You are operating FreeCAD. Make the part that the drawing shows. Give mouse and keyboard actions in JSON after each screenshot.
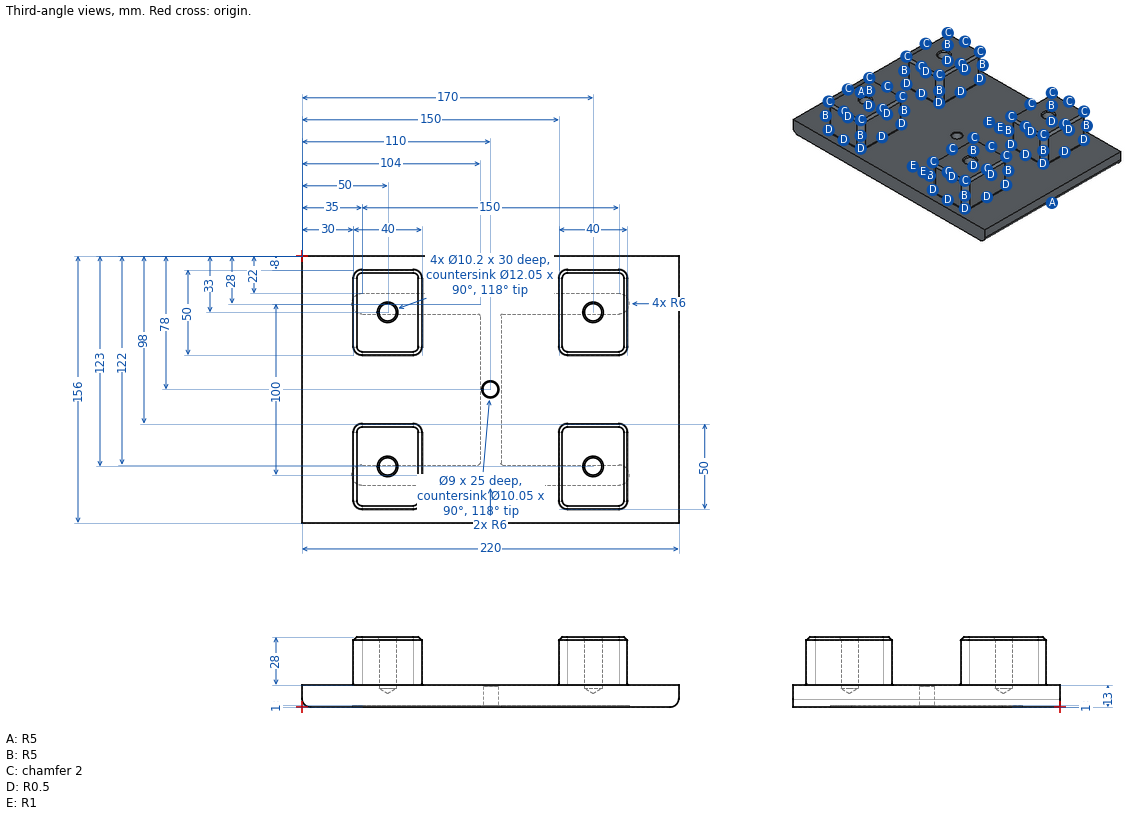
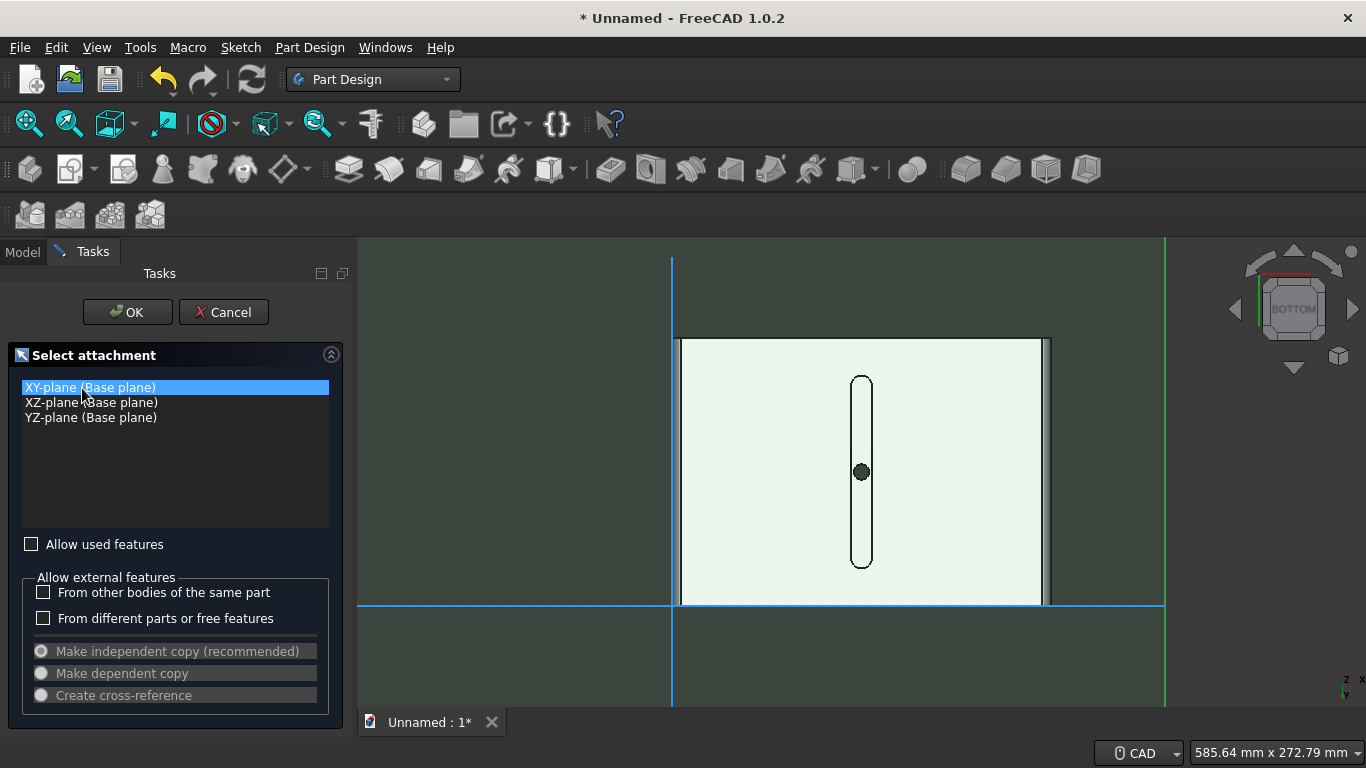
{"action": "left_click", "coordinate": [128, 312]}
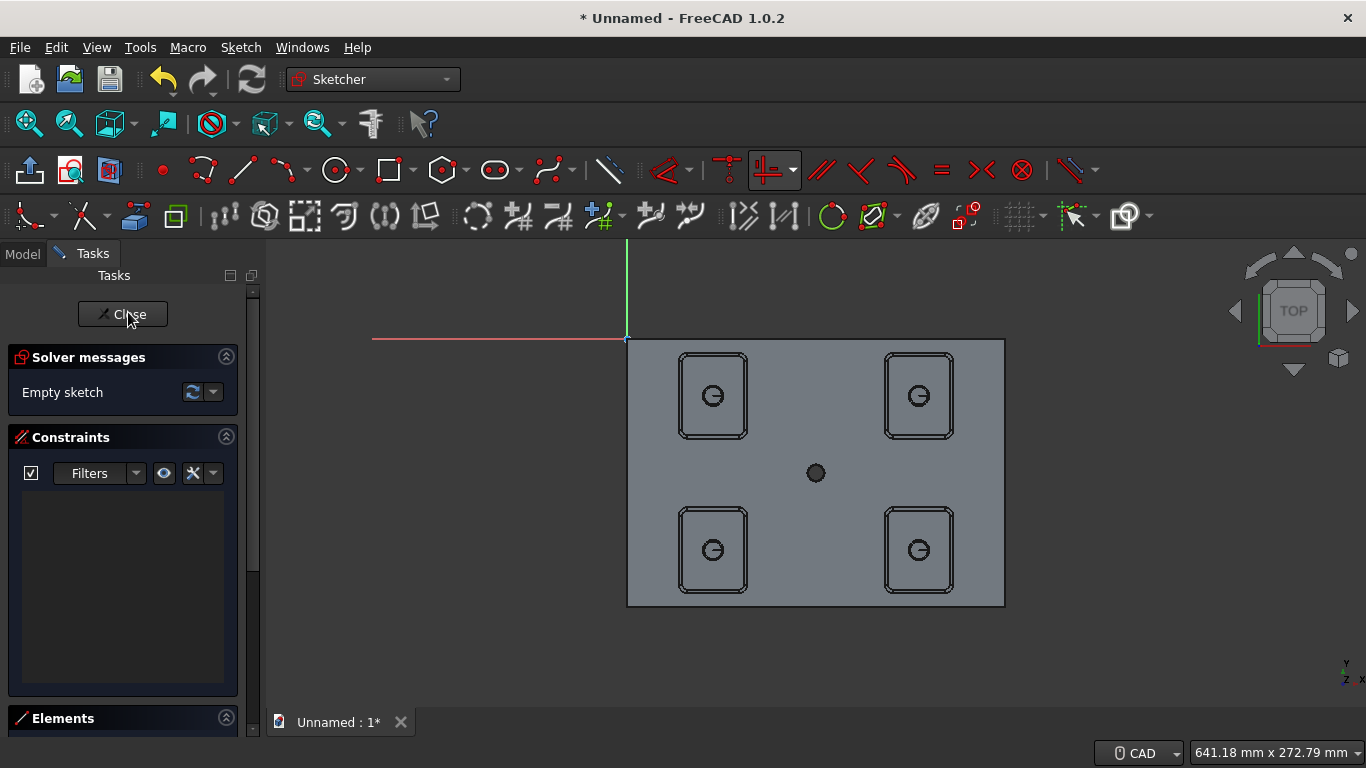
{"action": "left_click", "coordinate": [110, 170]}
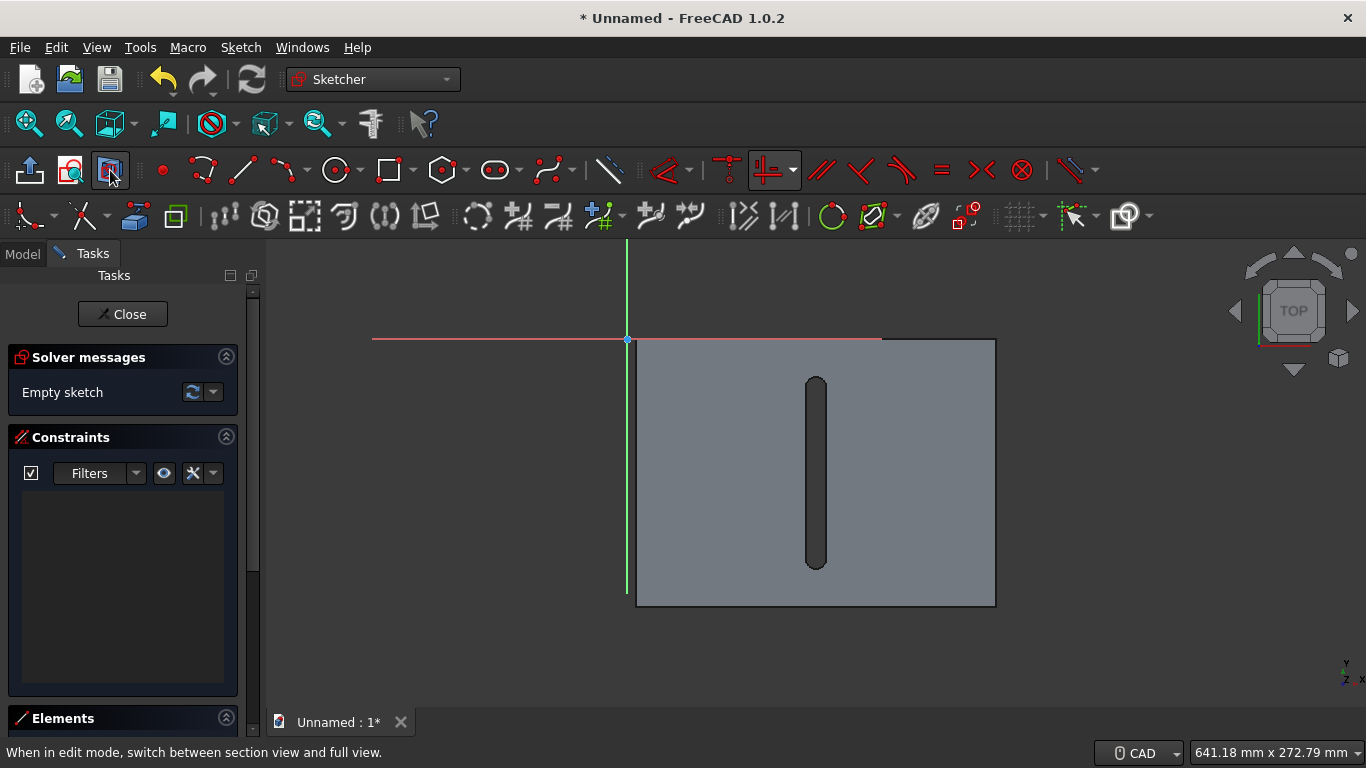
{"action": "key", "text": "g s"}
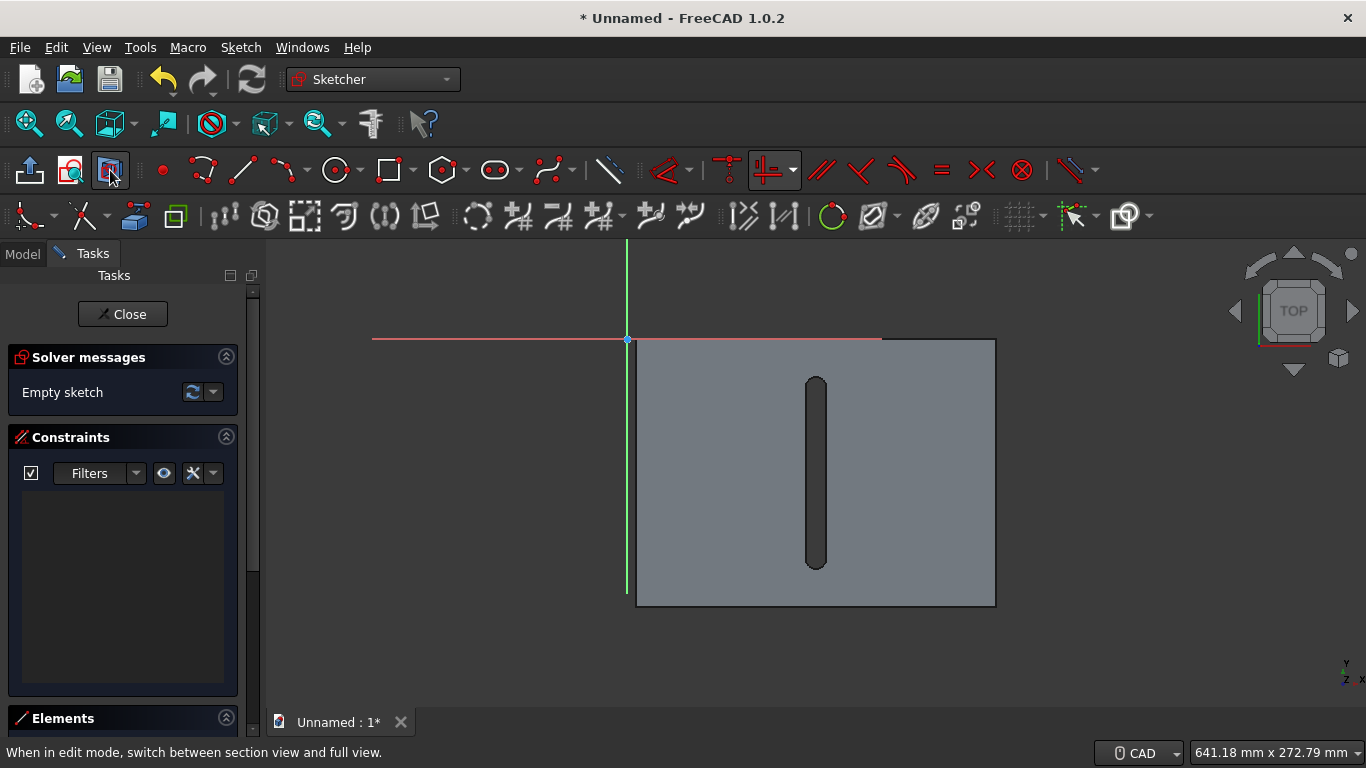
{"action": "scroll", "coordinate": [687, 387], "scroll_direction": "up", "scroll_amount": 4}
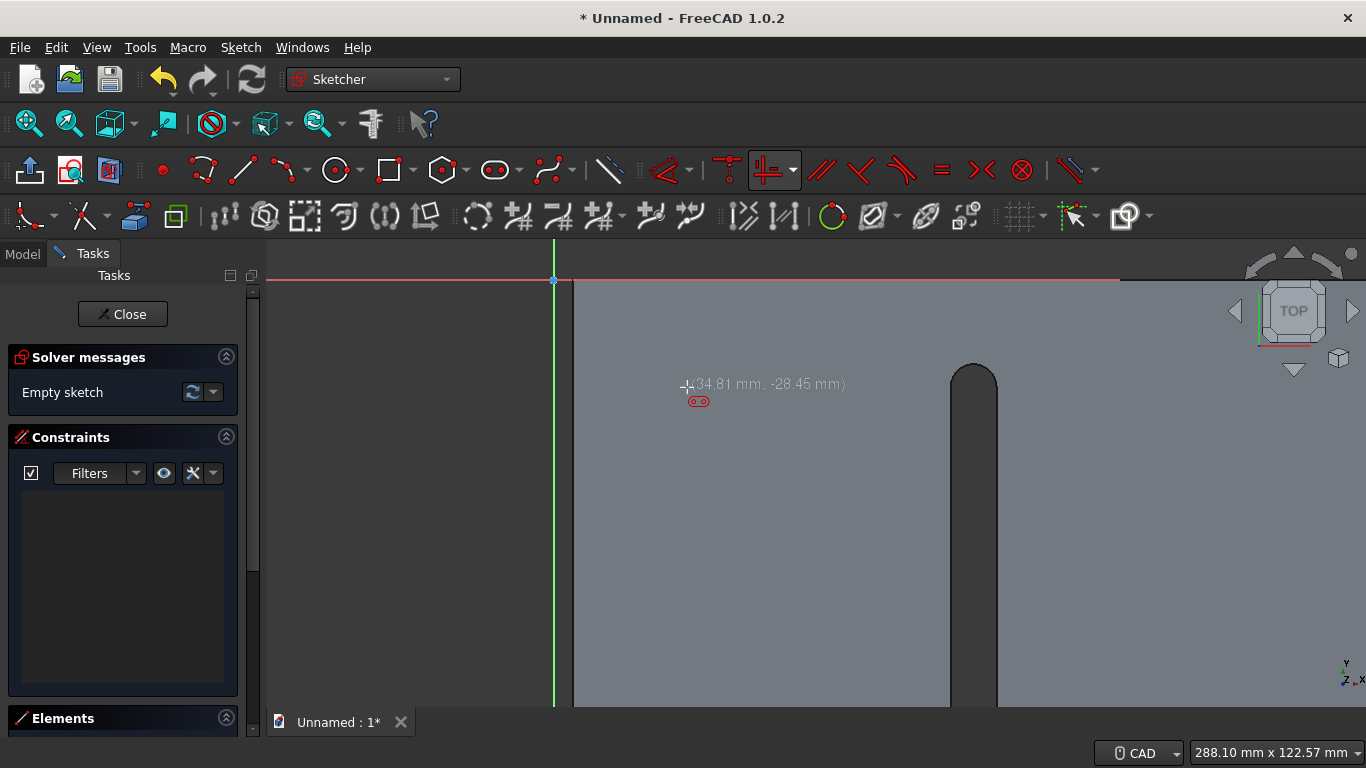
{"action": "left_click", "coordinate": [687, 387]}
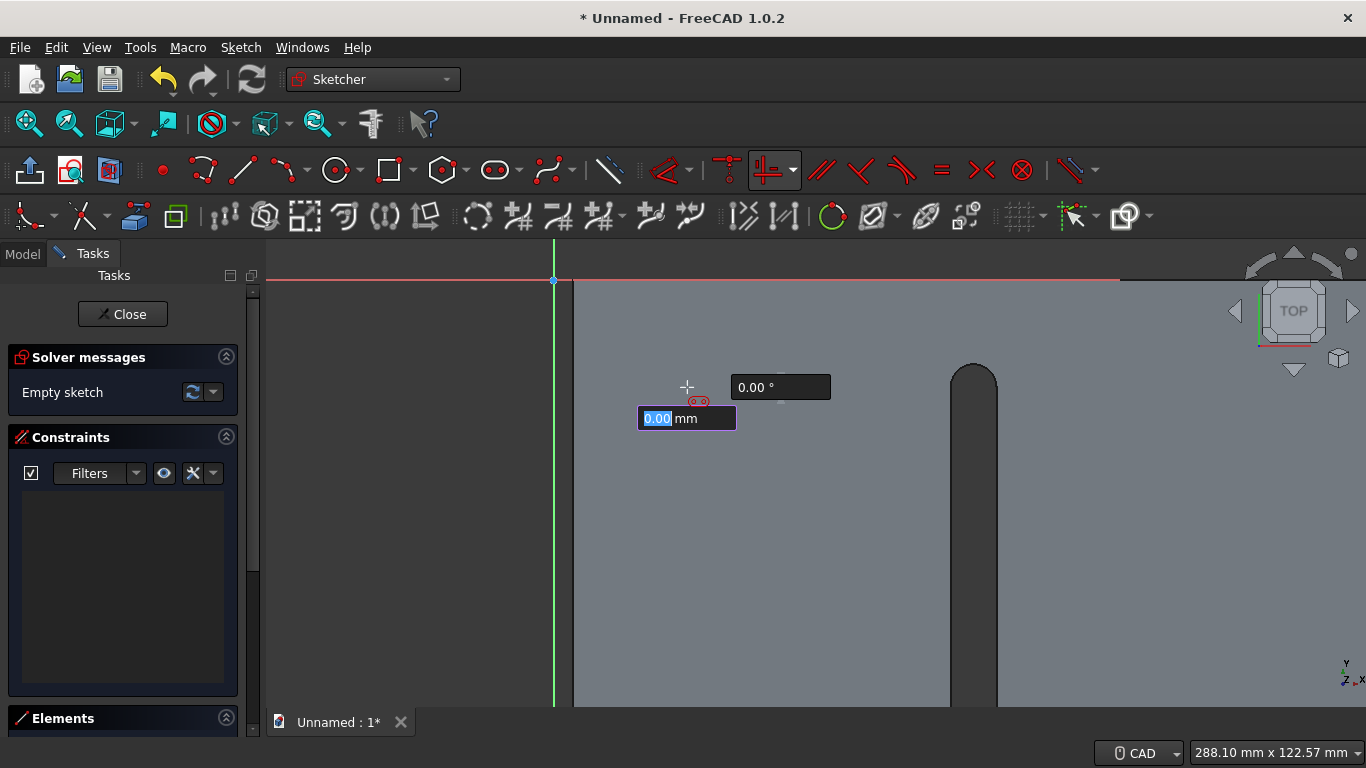
{"action": "scroll", "coordinate": [540, 396], "scroll_direction": "down", "scroll_amount": 3}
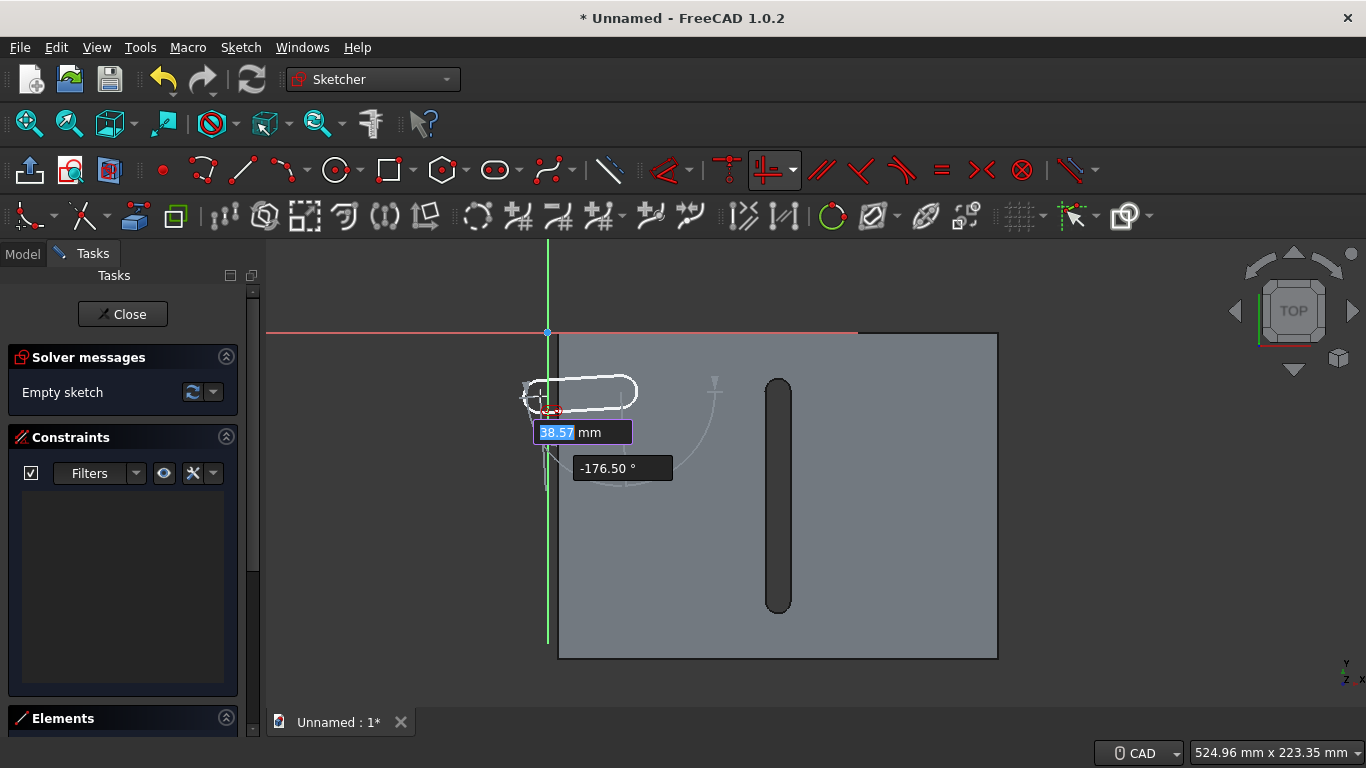
{"action": "left_click", "coordinate": [935, 391]}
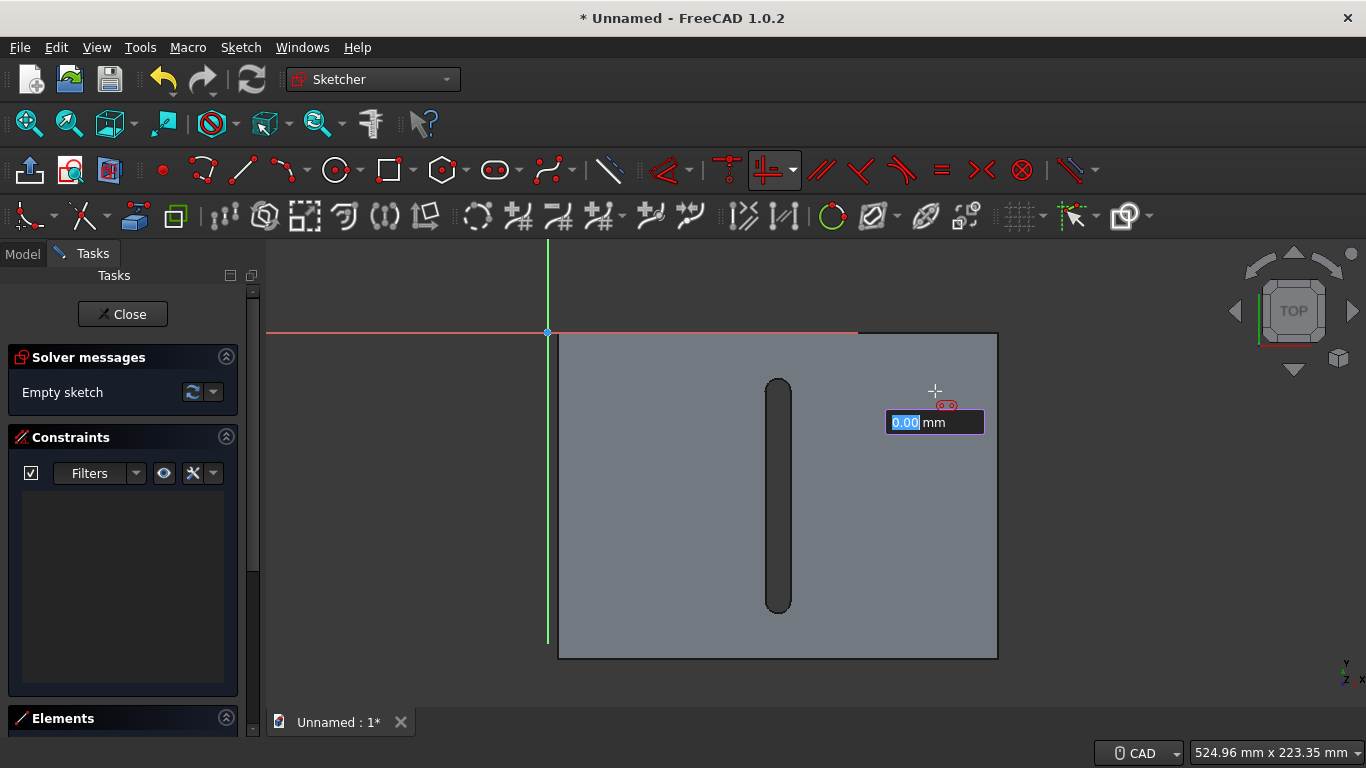
{"action": "scroll", "coordinate": [778, 379], "scroll_direction": "up", "scroll_amount": 2}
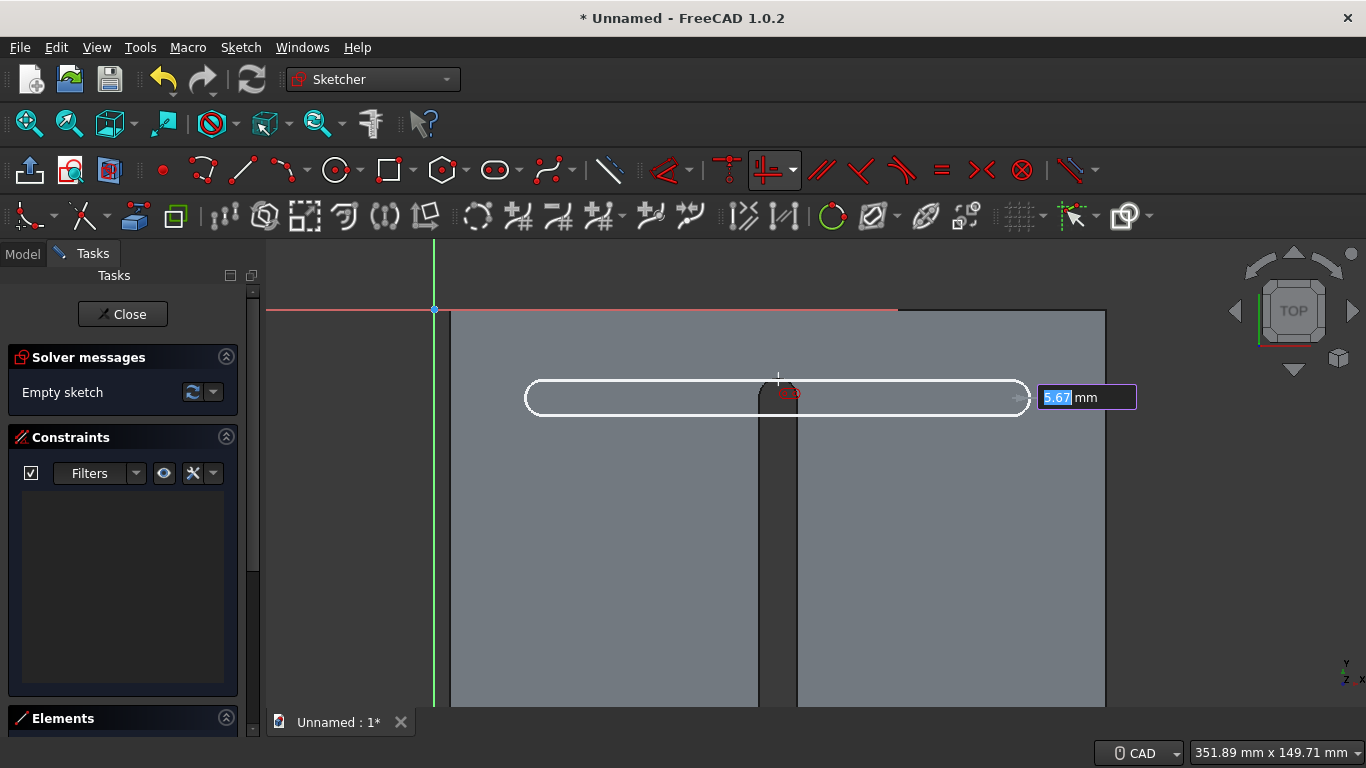
{"action": "left_click", "coordinate": [778, 378]}